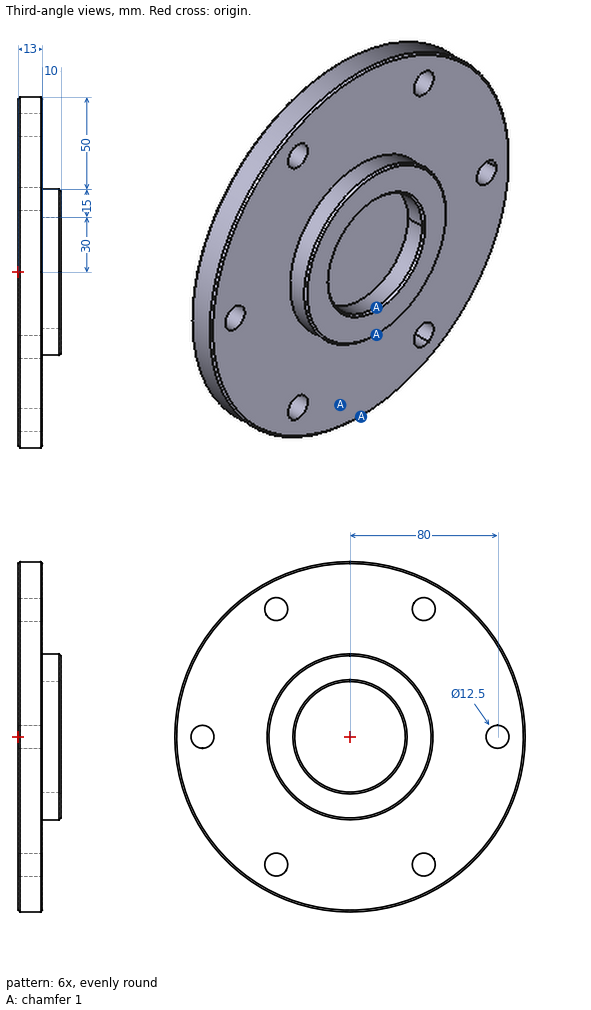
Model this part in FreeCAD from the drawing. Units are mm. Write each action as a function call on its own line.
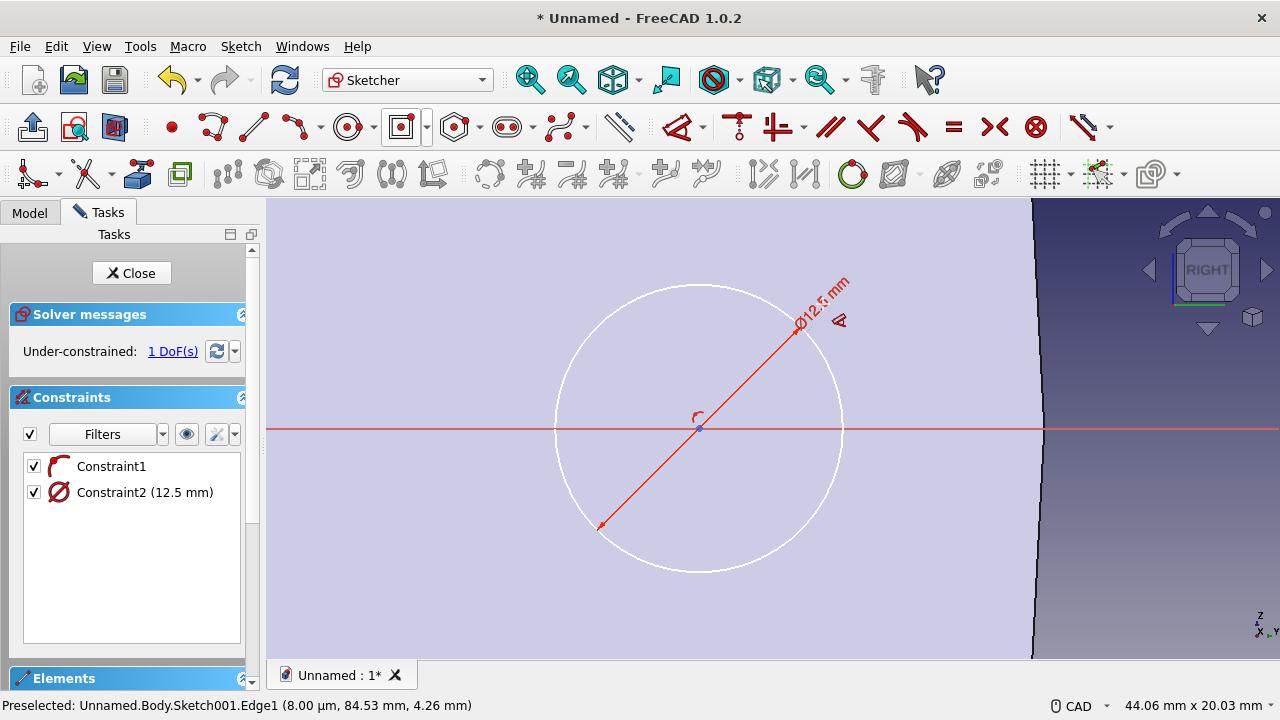
click(699, 428)
click(496, 462)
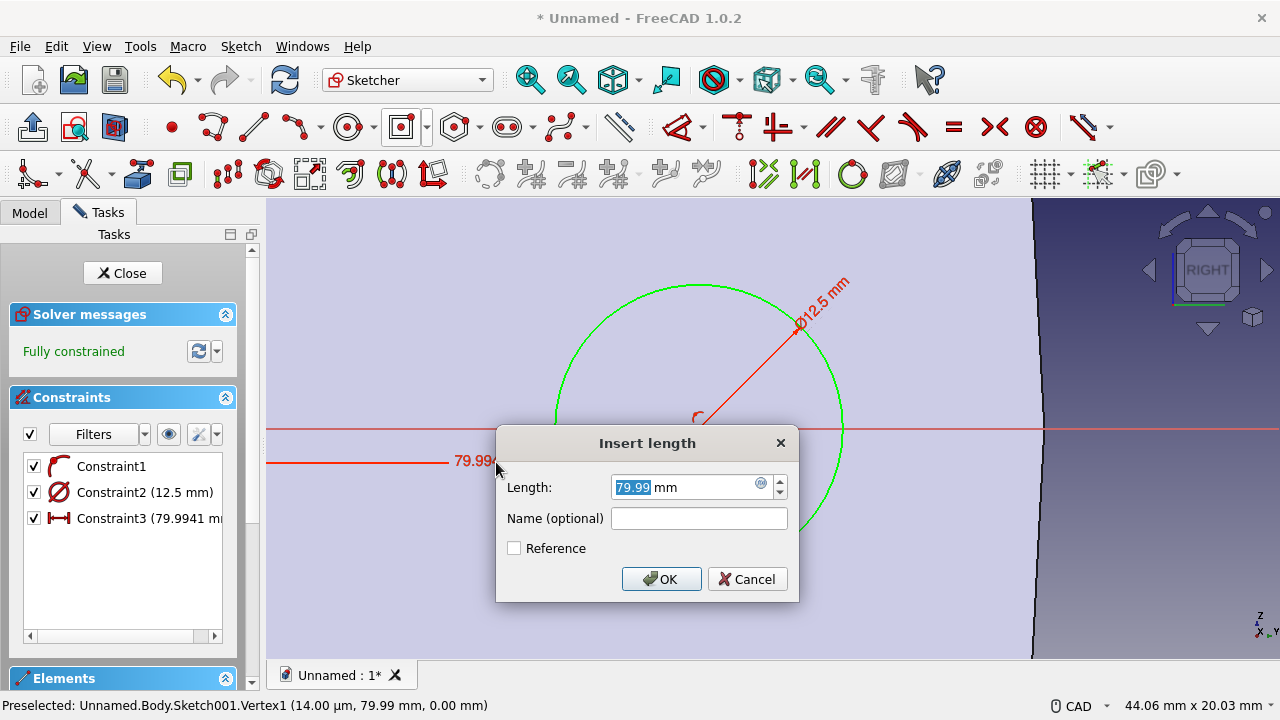
text(80)
key(Return)
key(Escape)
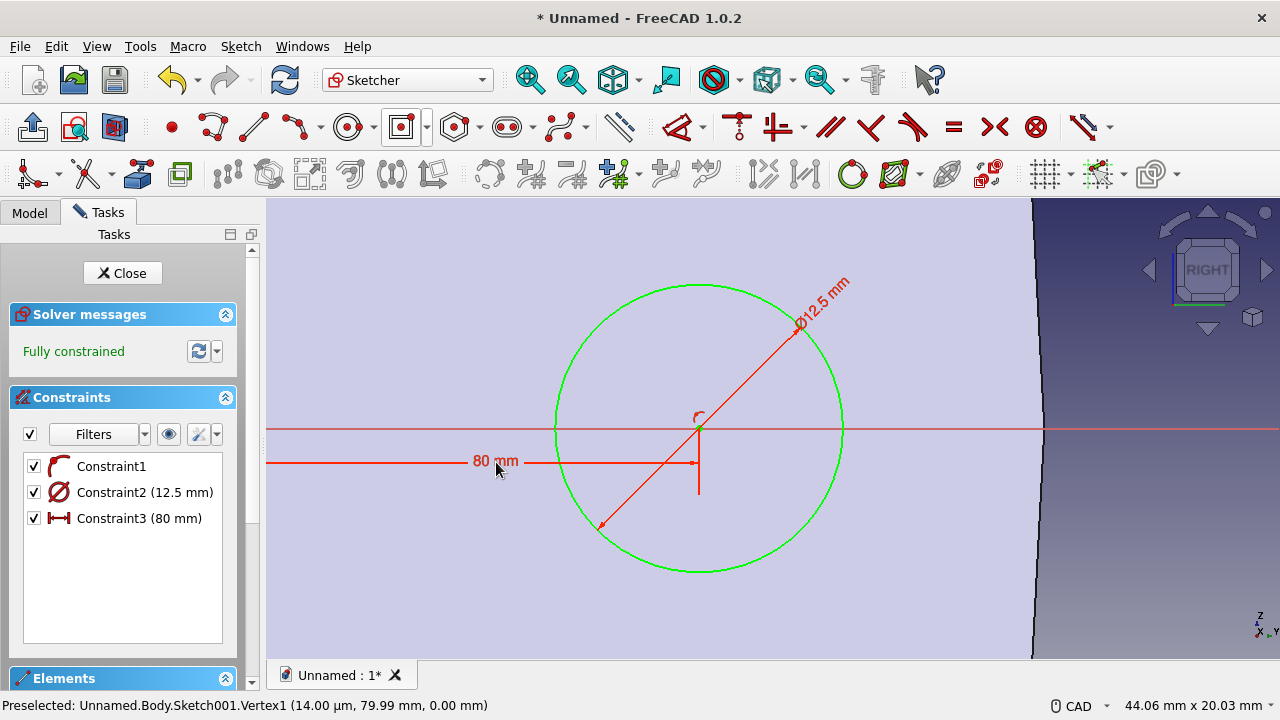
click(123, 273)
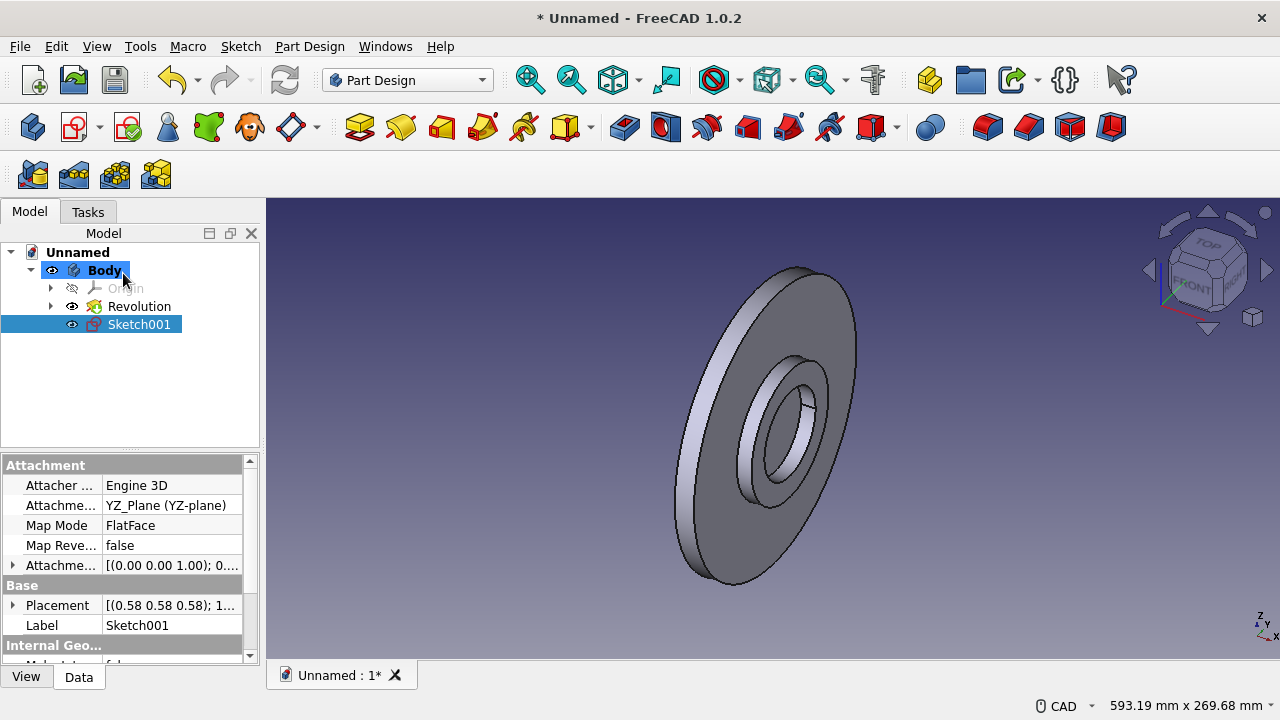
click(625, 128)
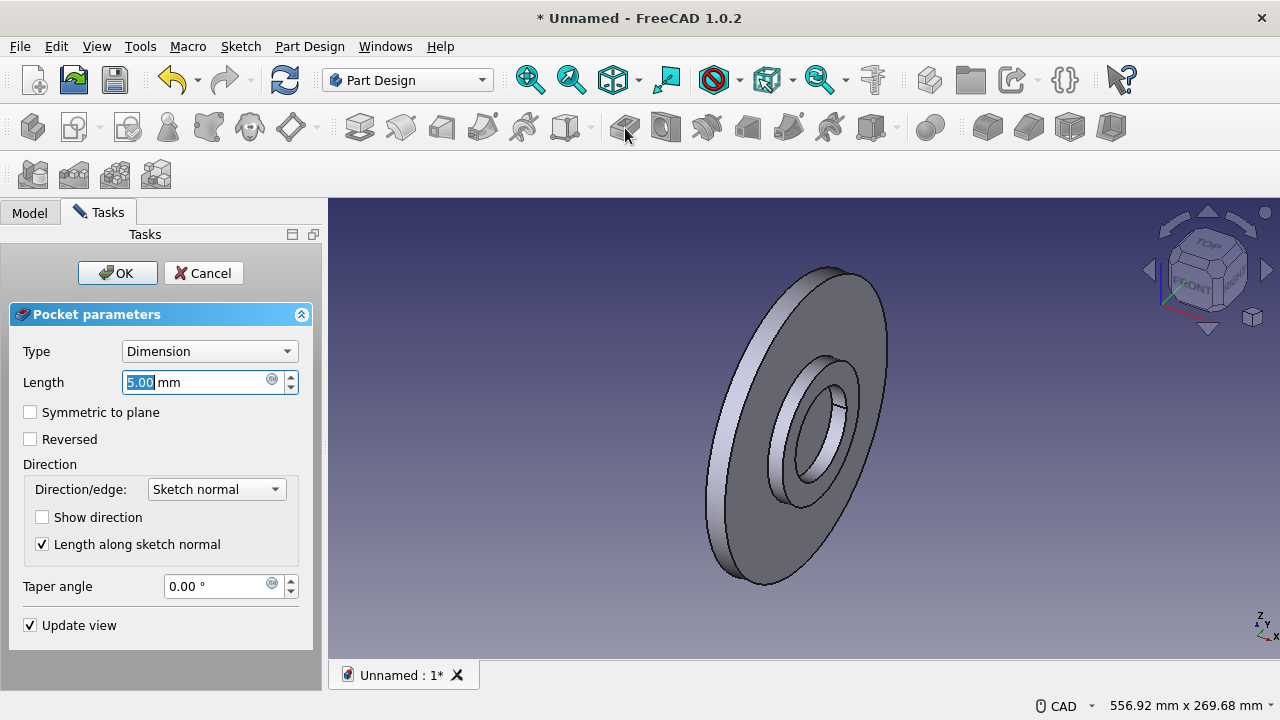
click(210, 352)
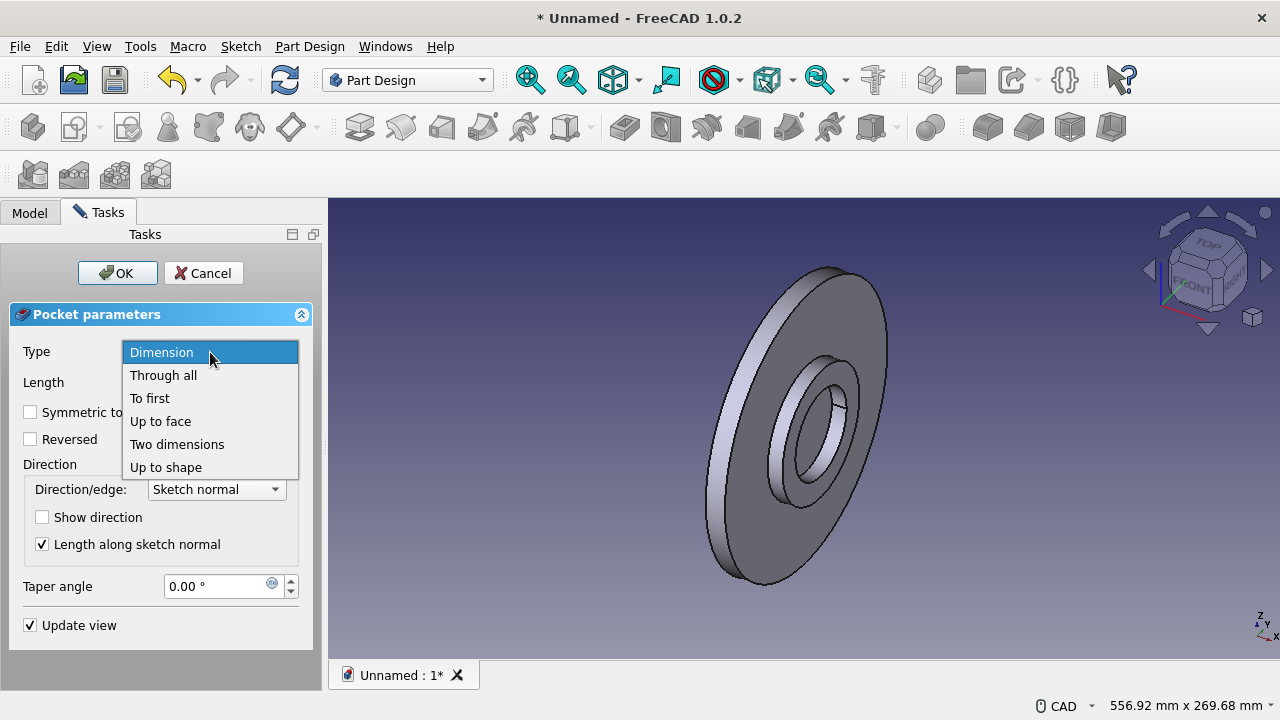
click(208, 376)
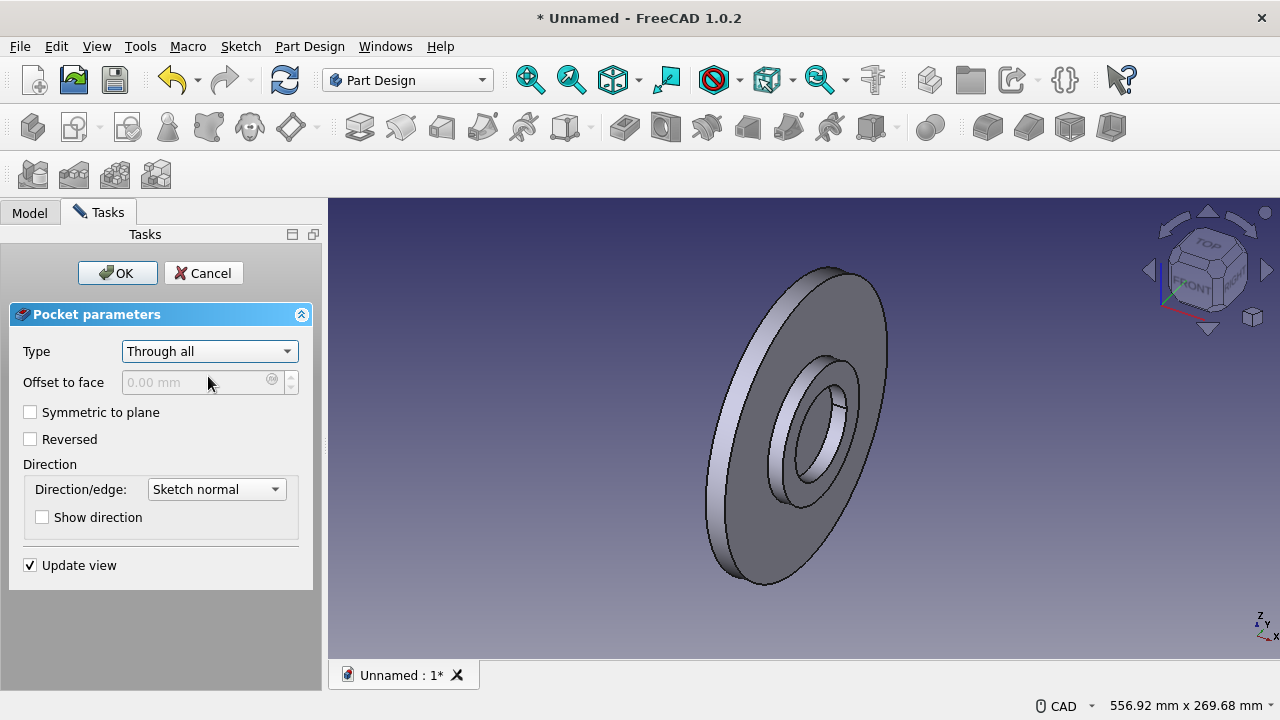
click(31, 439)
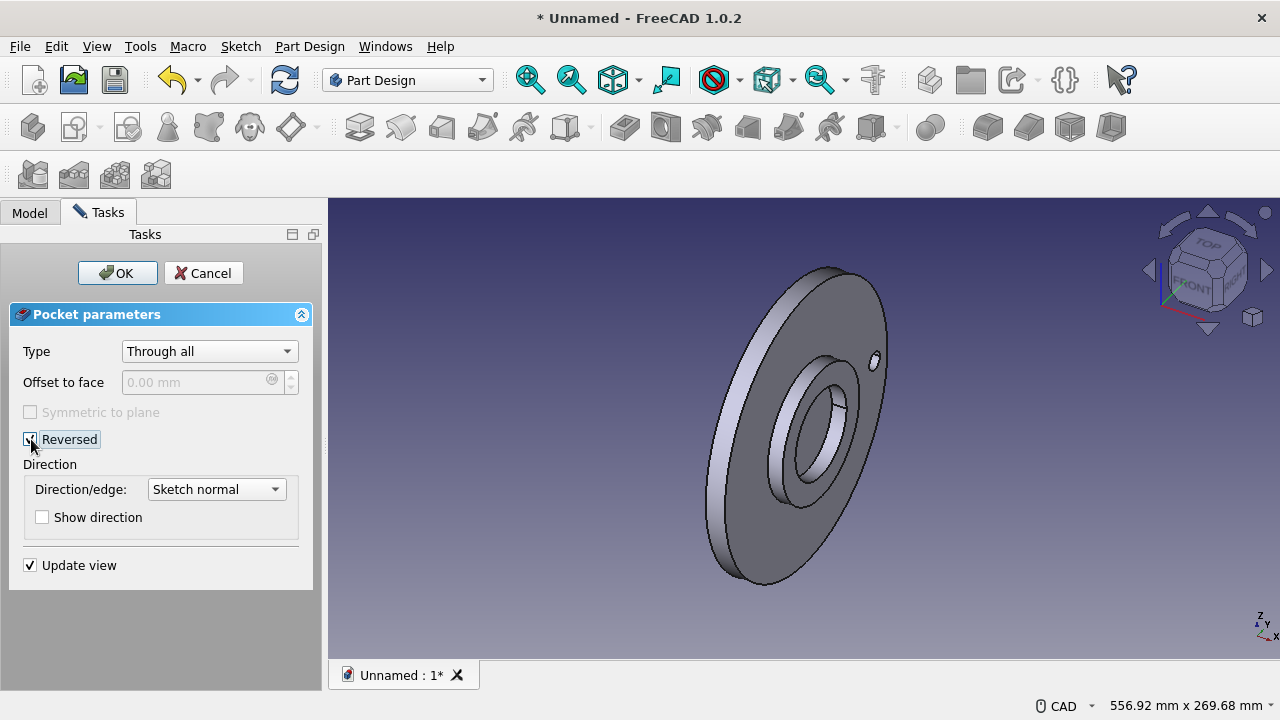
click(118, 273)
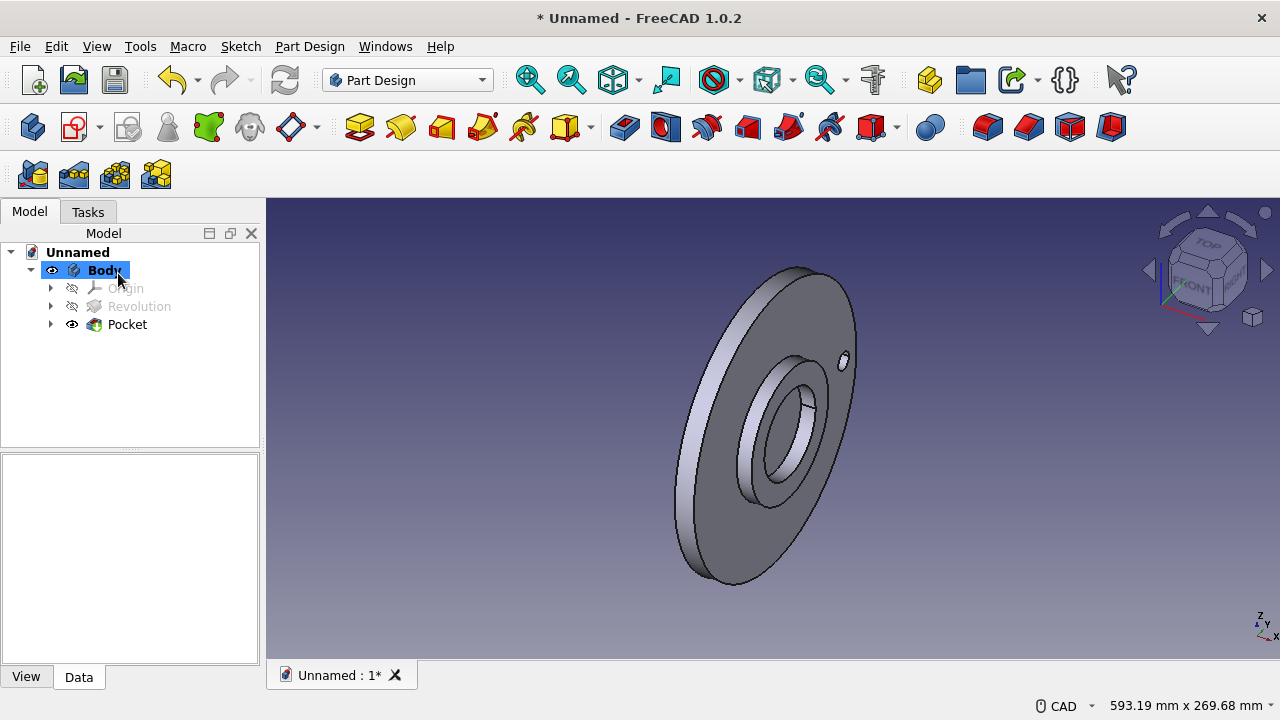
click(117, 324)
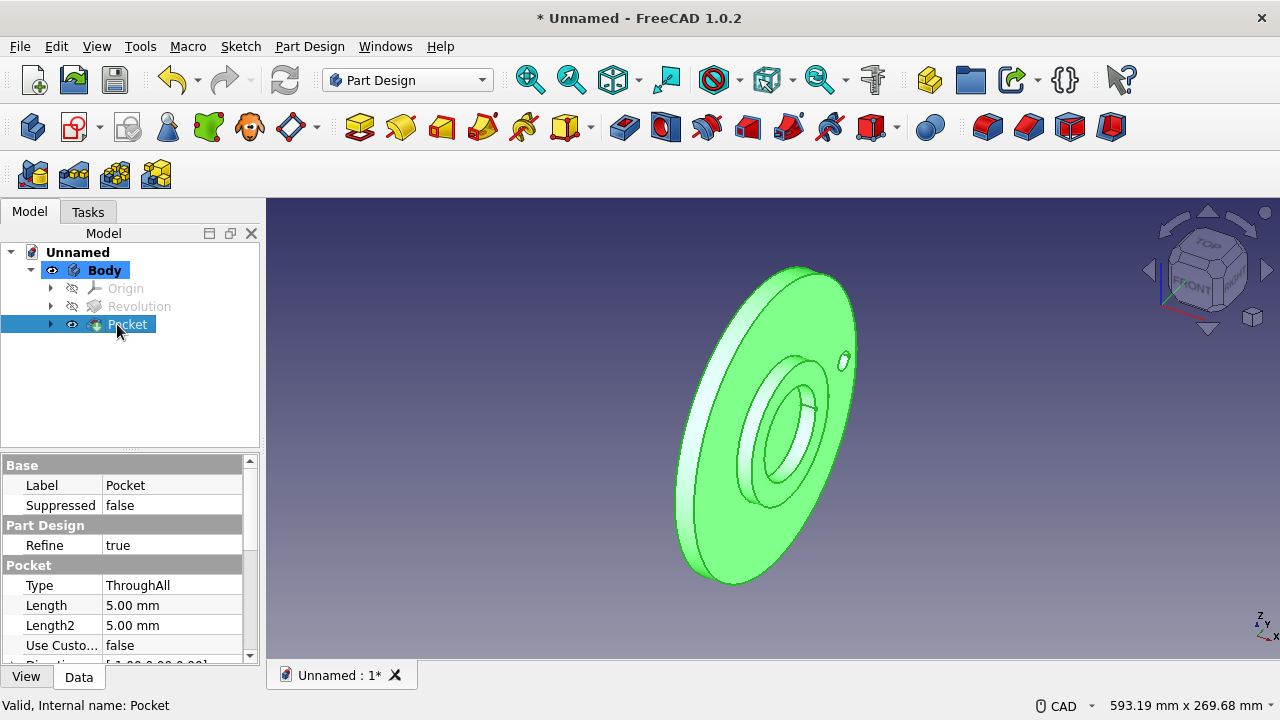
click(115, 174)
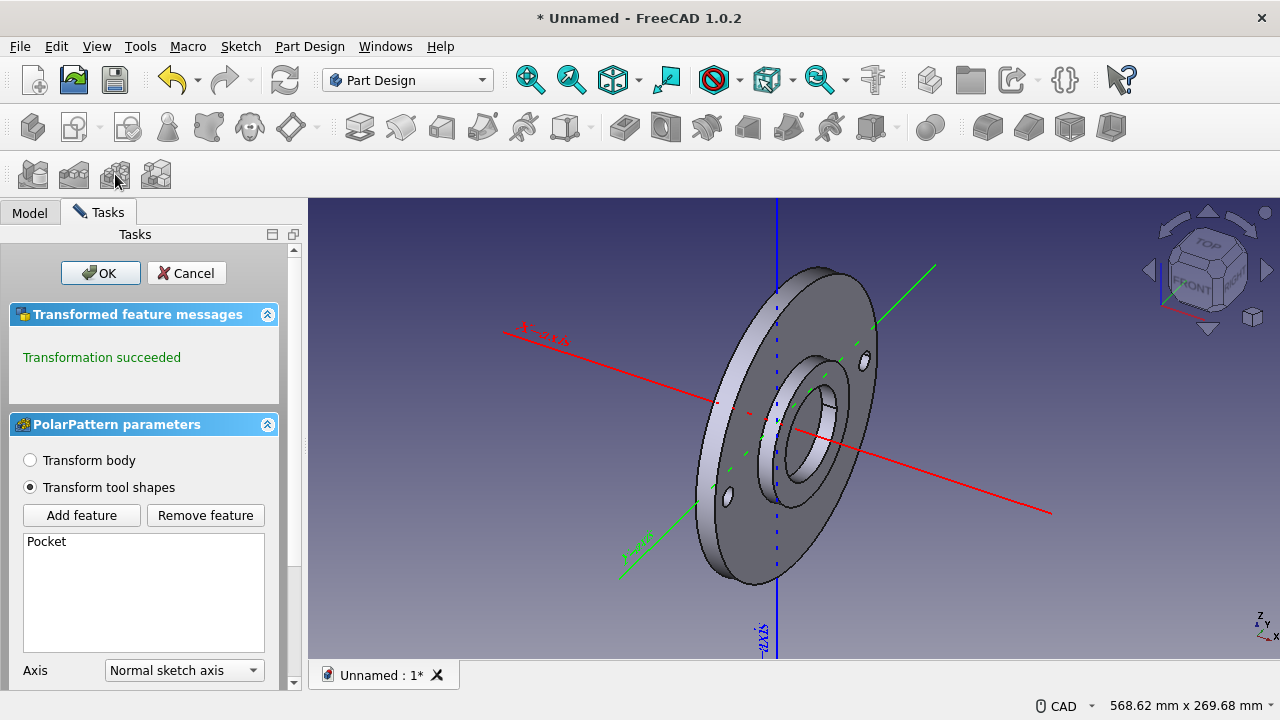
click(185, 670)